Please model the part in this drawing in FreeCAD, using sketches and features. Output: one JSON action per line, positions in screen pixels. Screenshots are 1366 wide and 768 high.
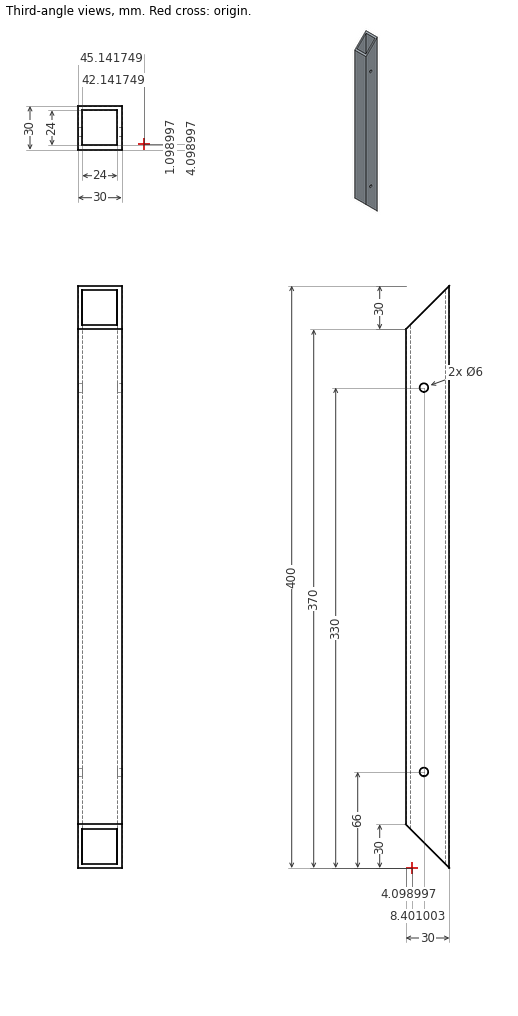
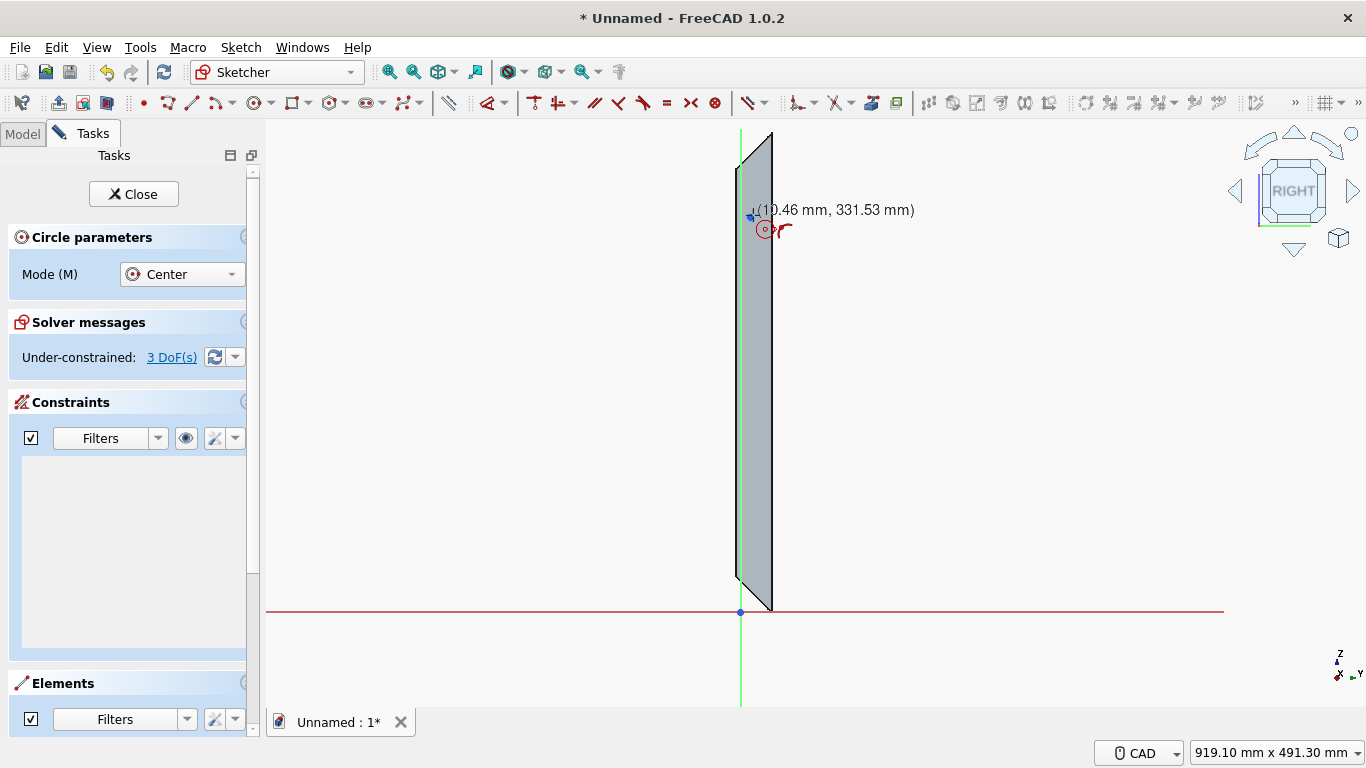
{"action": "scroll", "coordinate": [751, 533], "scroll_direction": "up", "scroll_amount": 10}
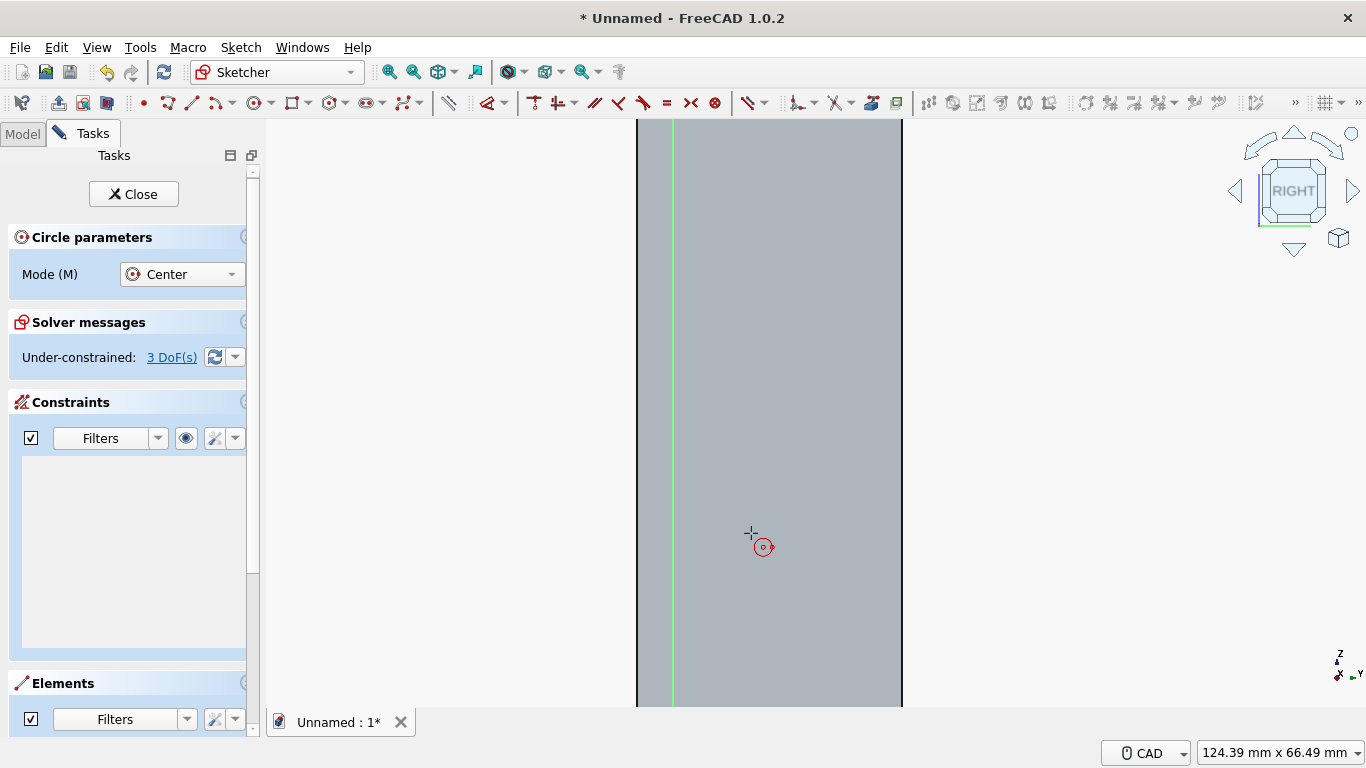
{"action": "scroll", "coordinate": [751, 534], "scroll_direction": "down", "scroll_amount": 10}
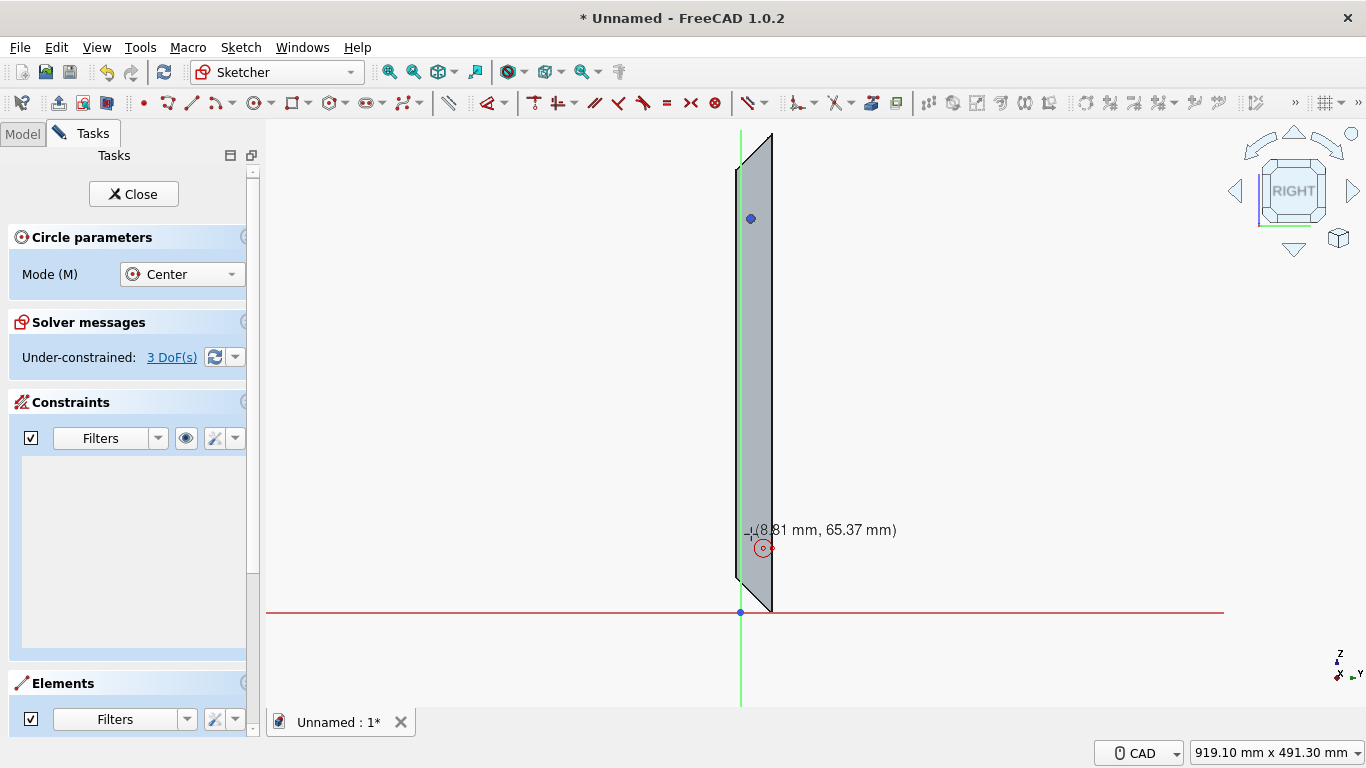
{"action": "scroll", "coordinate": [751, 534], "scroll_direction": "up", "scroll_amount": 3}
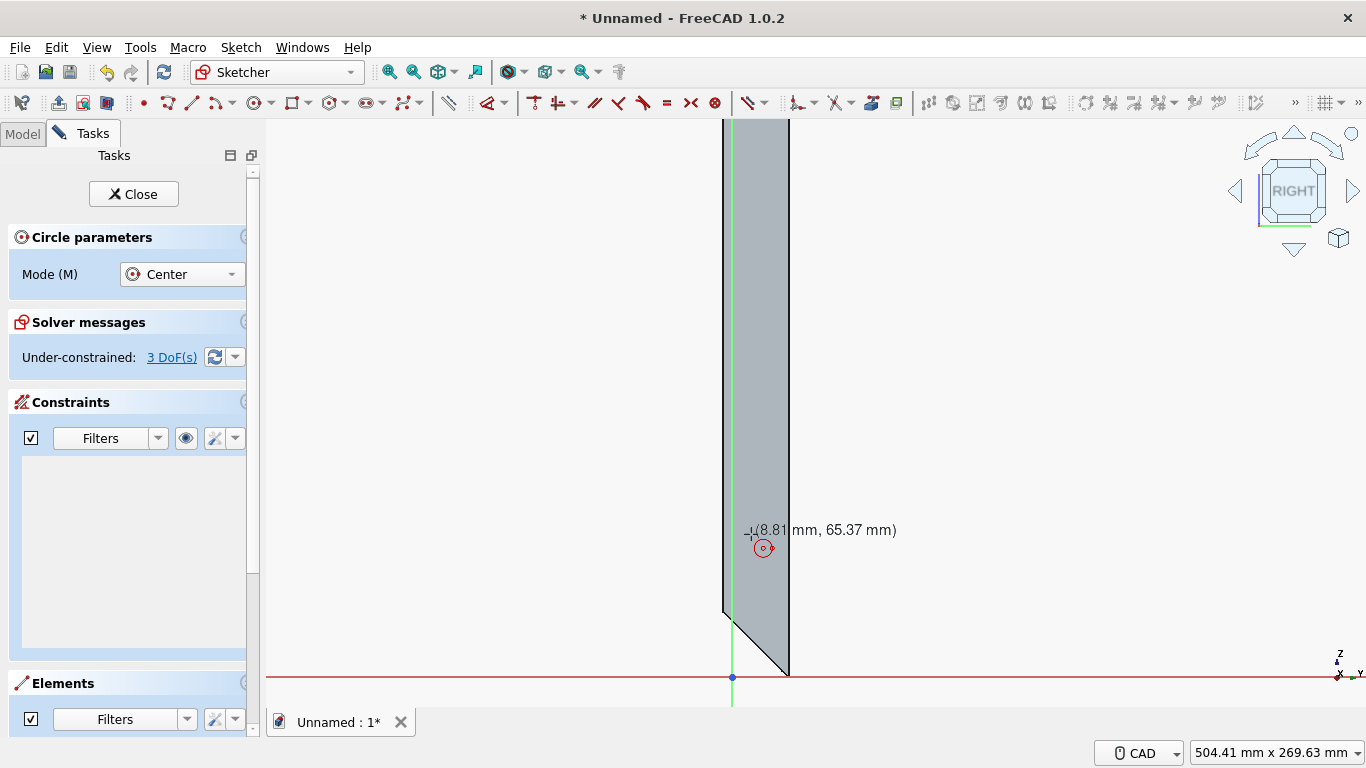
{"action": "left_click", "coordinate": [750, 533]}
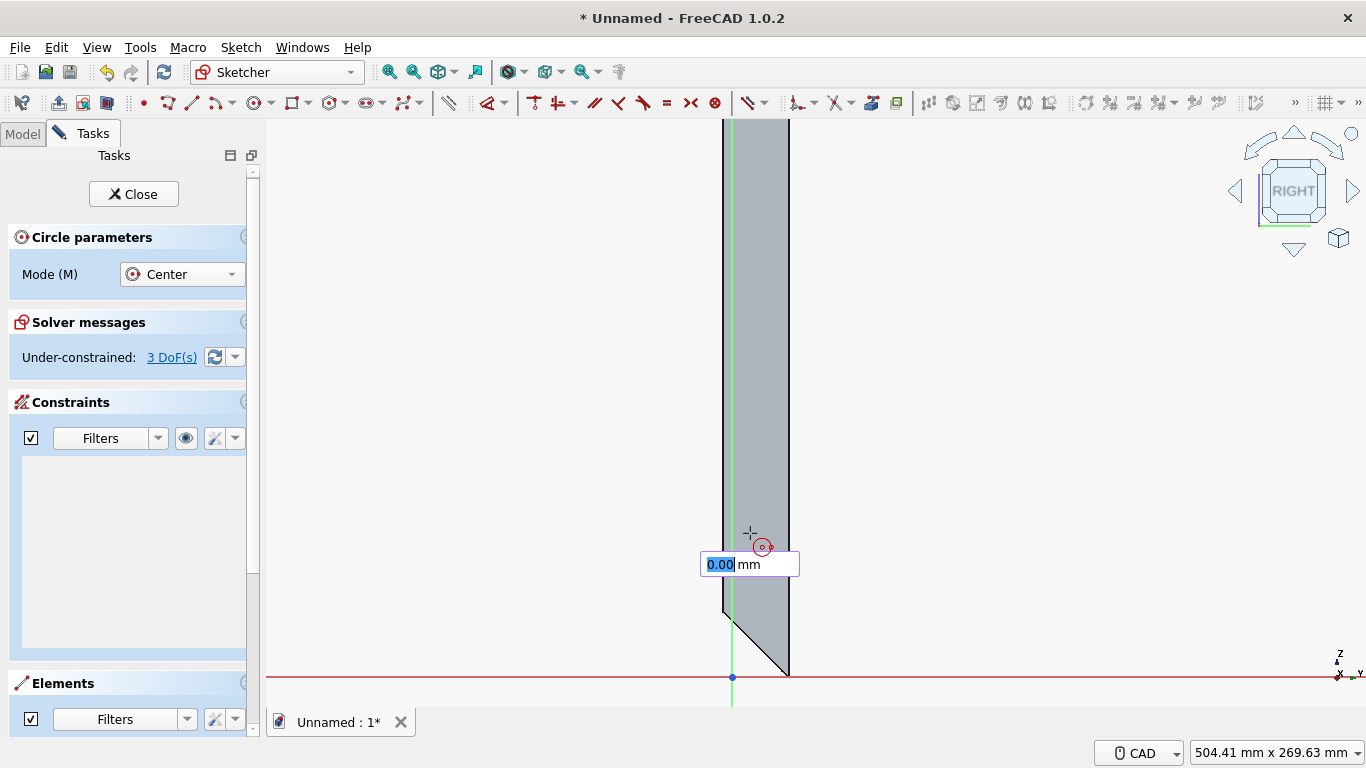
{"action": "scroll", "coordinate": [755, 529], "scroll_direction": "up", "scroll_amount": 5}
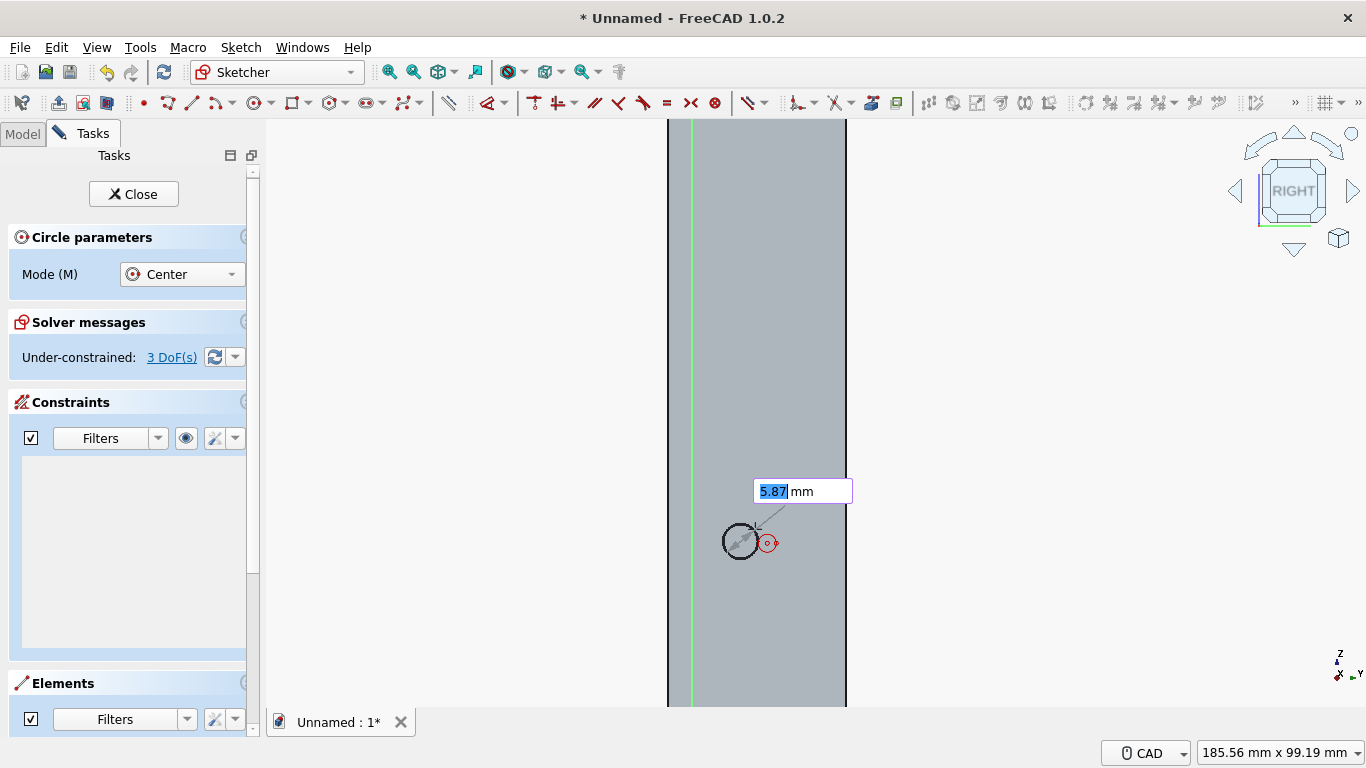
{"action": "left_click", "coordinate": [754, 527]}
{"action": "key", "text": "Escape"}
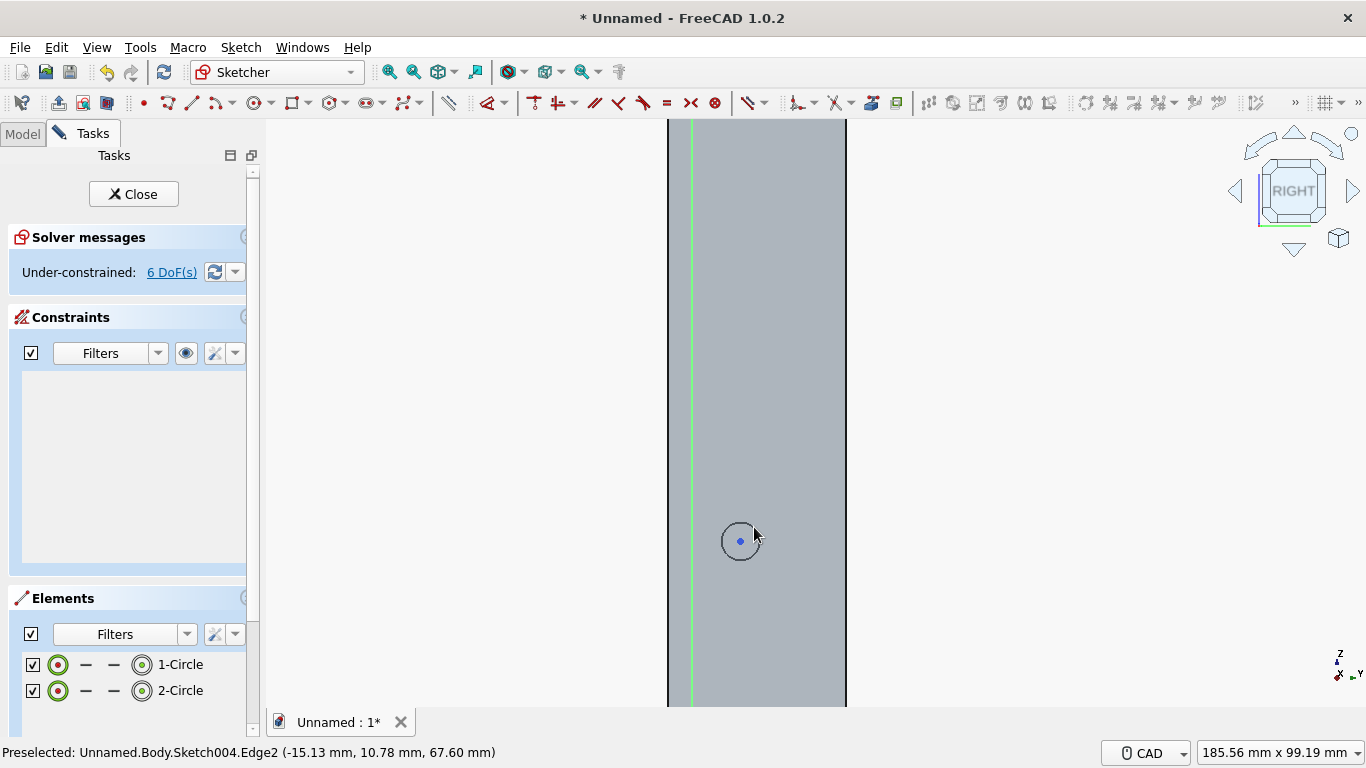
{"action": "scroll", "coordinate": [753, 532], "scroll_direction": "down", "scroll_amount": 8}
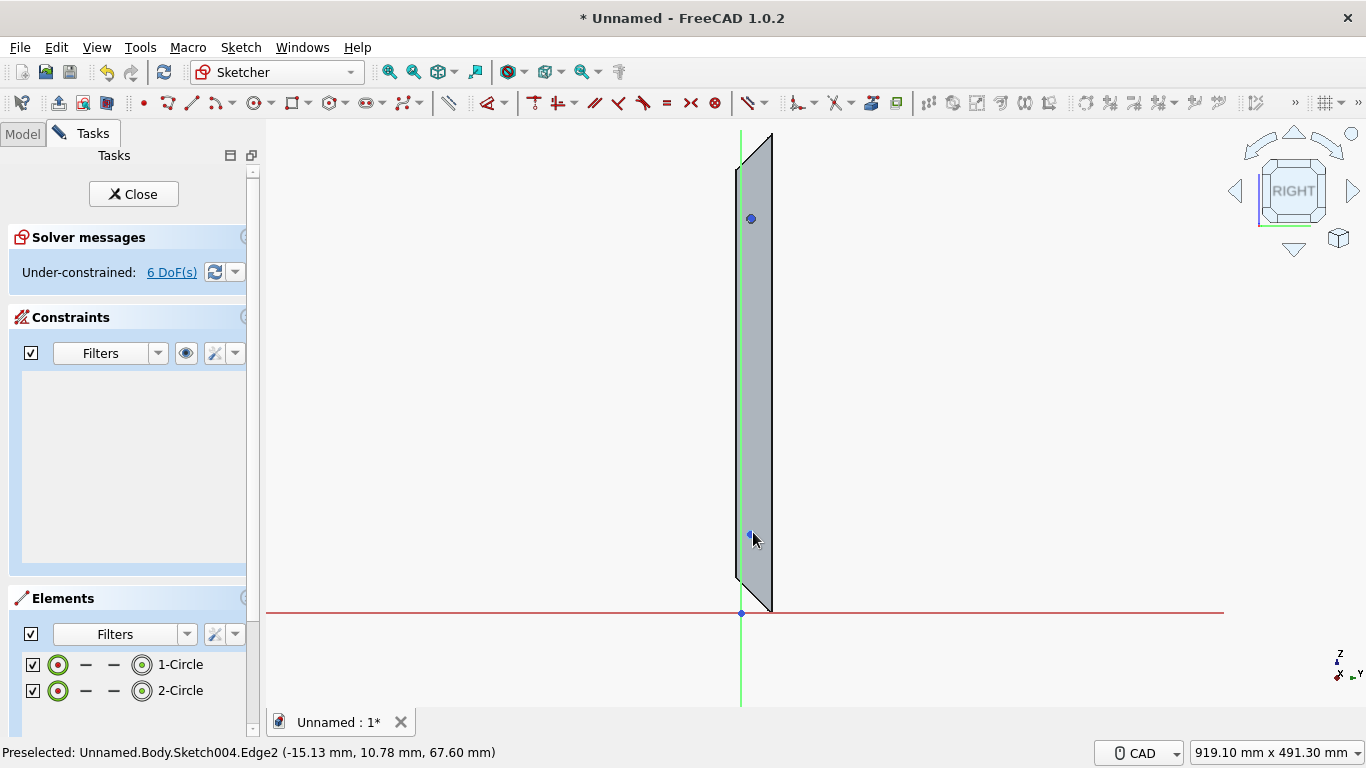
{"action": "scroll", "coordinate": [754, 216], "scroll_direction": "up", "scroll_amount": 7}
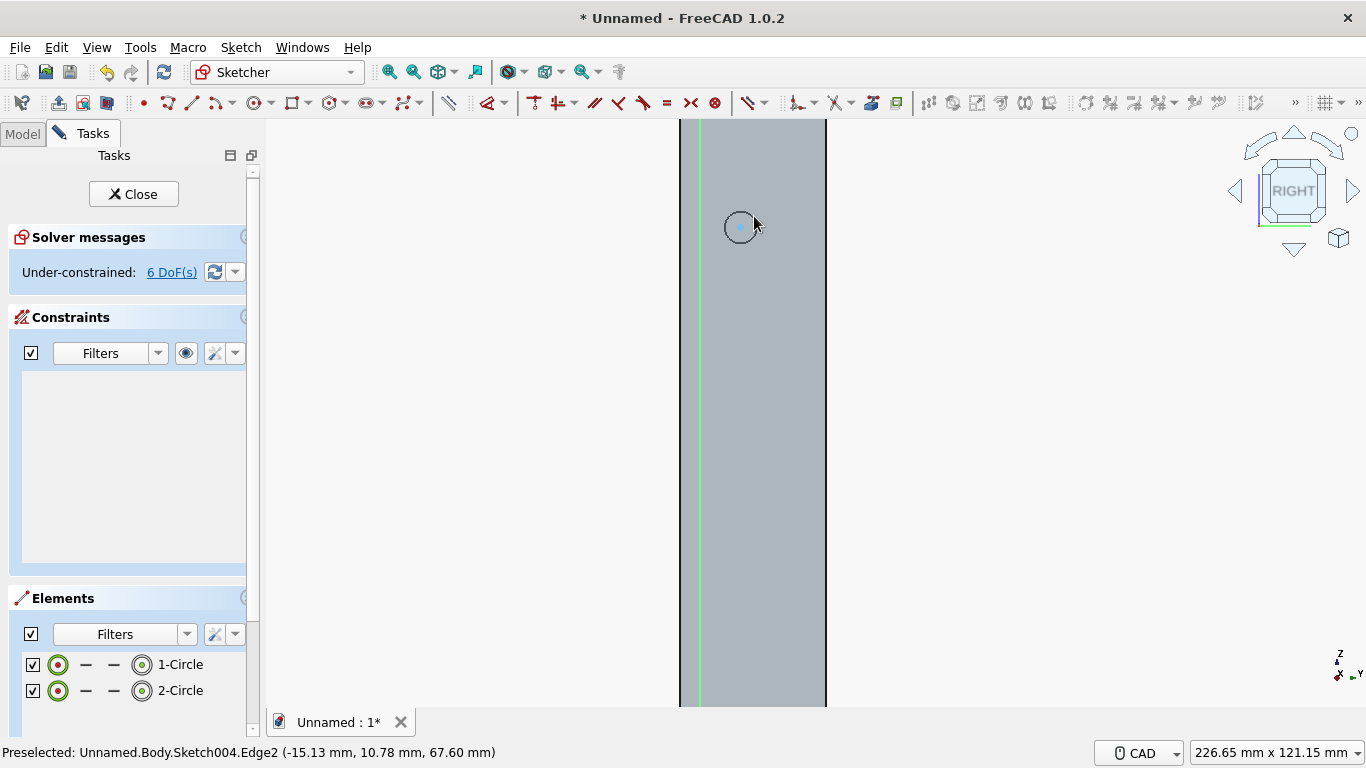
{"action": "left_click", "coordinate": [752, 216]}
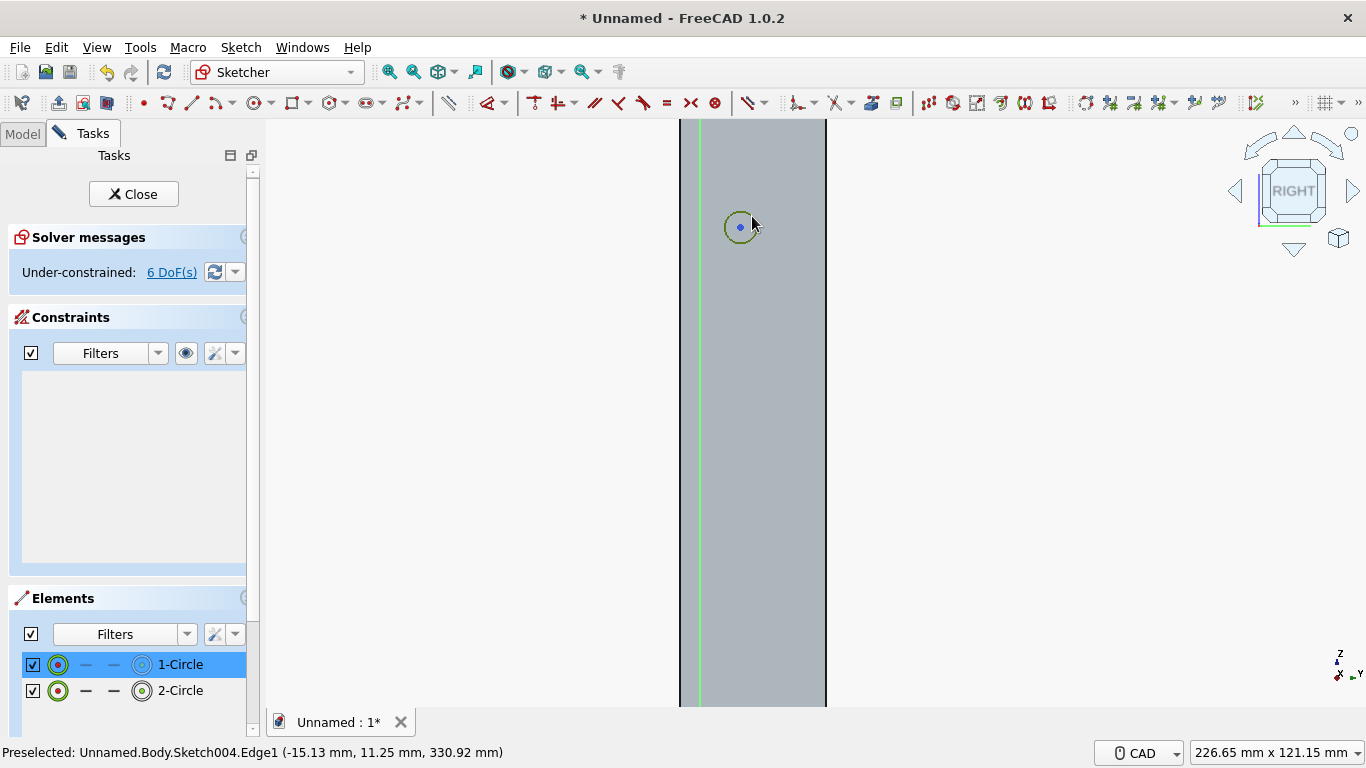
{"action": "scroll", "coordinate": [754, 215], "scroll_direction": "down", "scroll_amount": 7}